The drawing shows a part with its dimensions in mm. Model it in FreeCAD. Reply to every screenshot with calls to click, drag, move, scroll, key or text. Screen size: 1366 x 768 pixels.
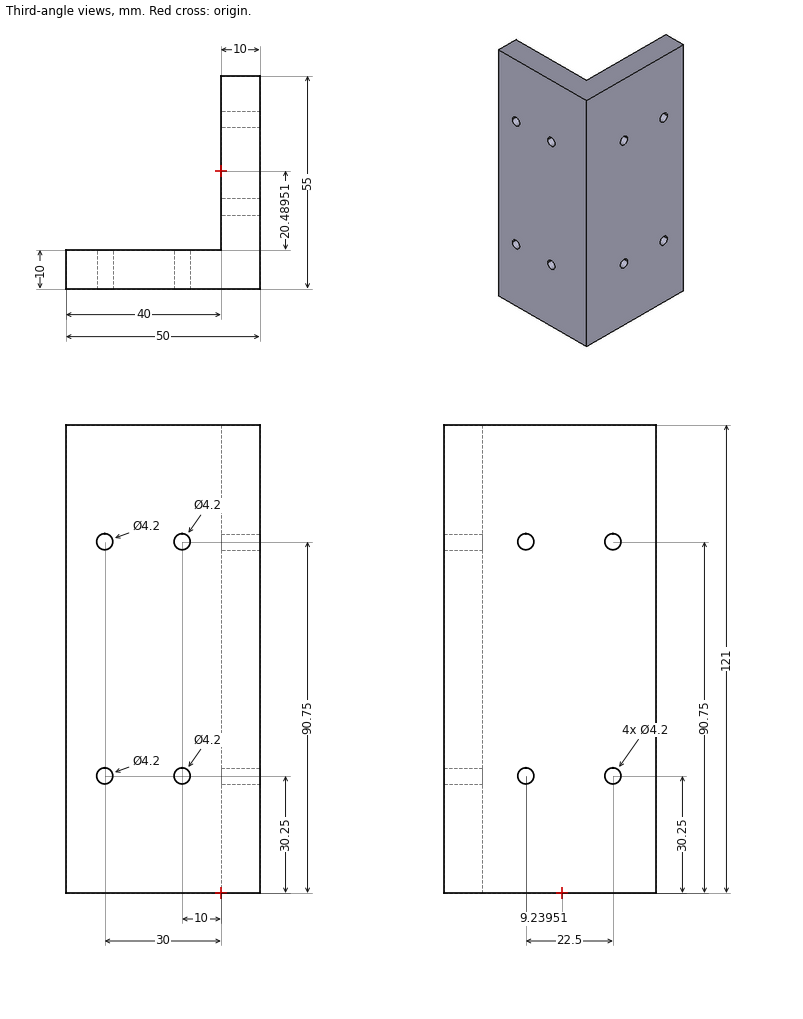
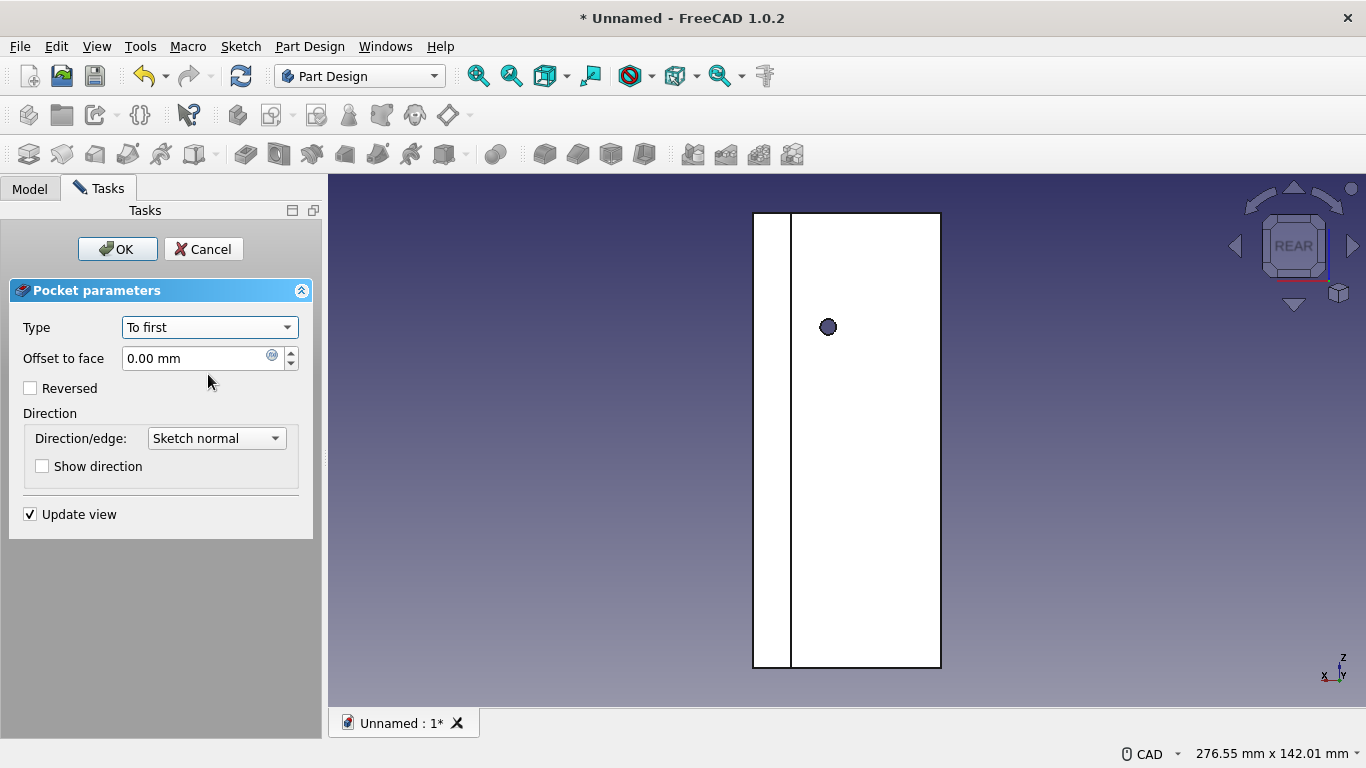
click(118, 249)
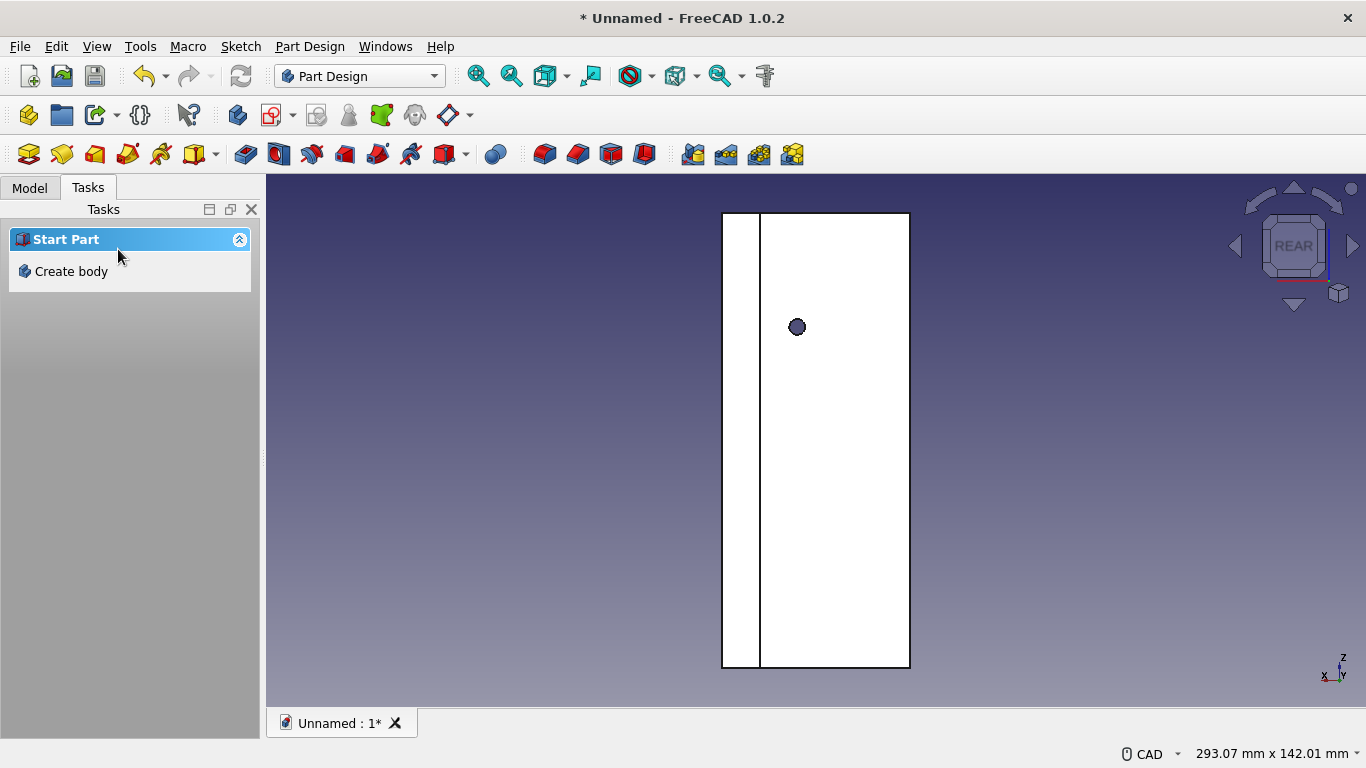
click(835, 439)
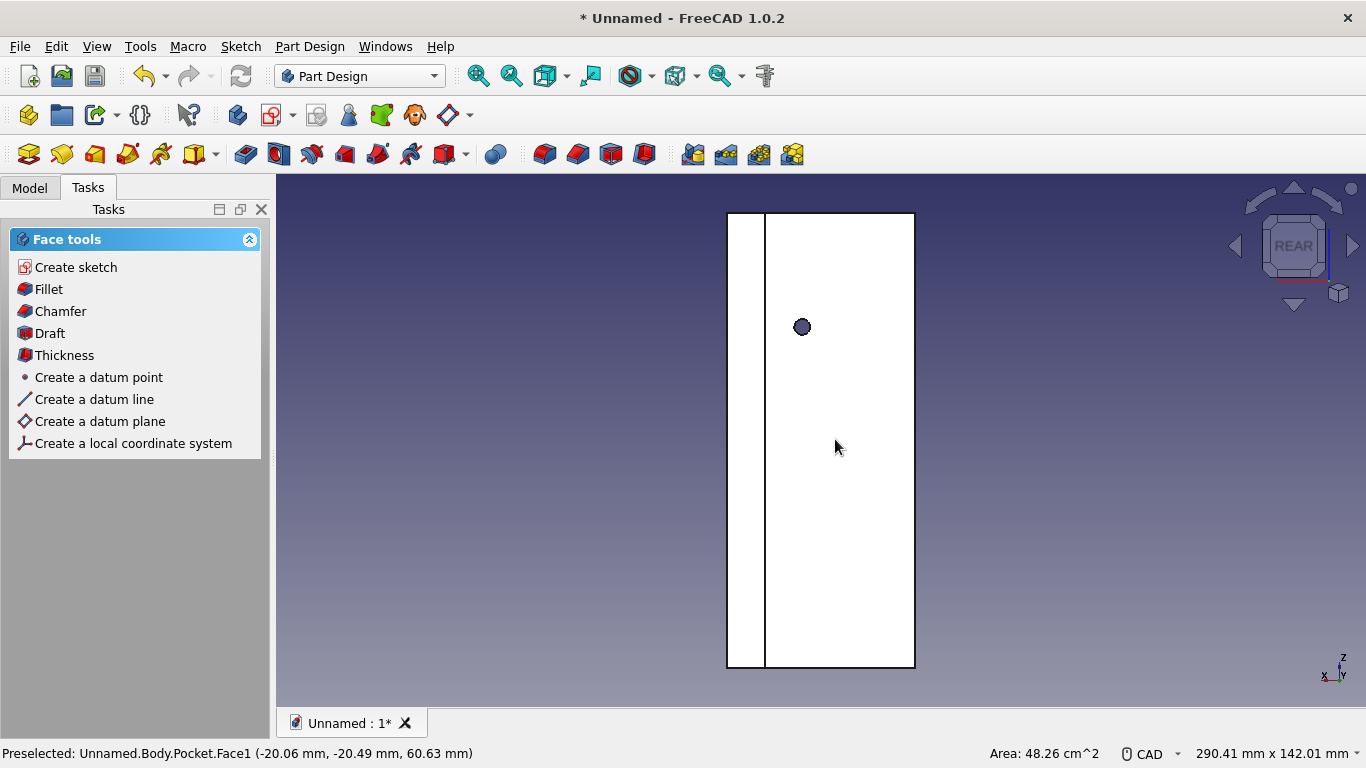
click(270, 116)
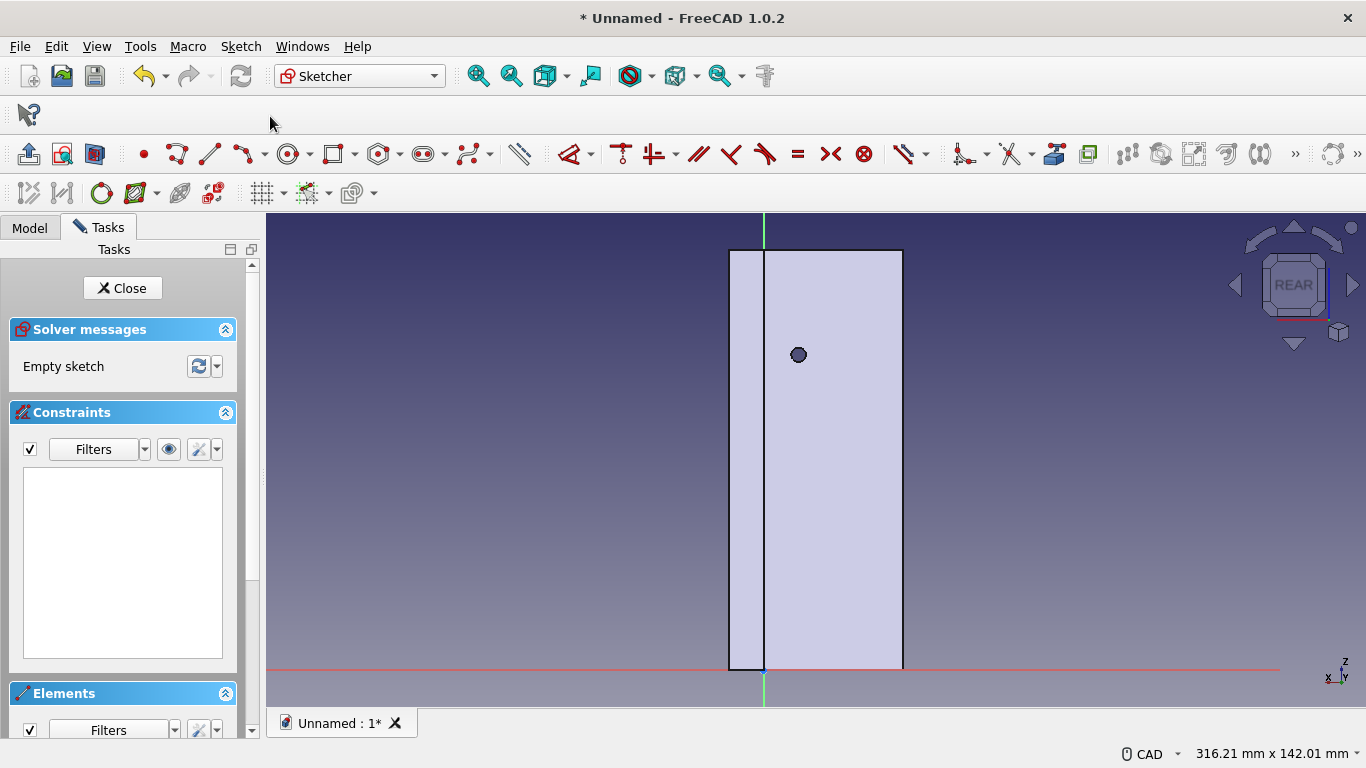
click(95, 154)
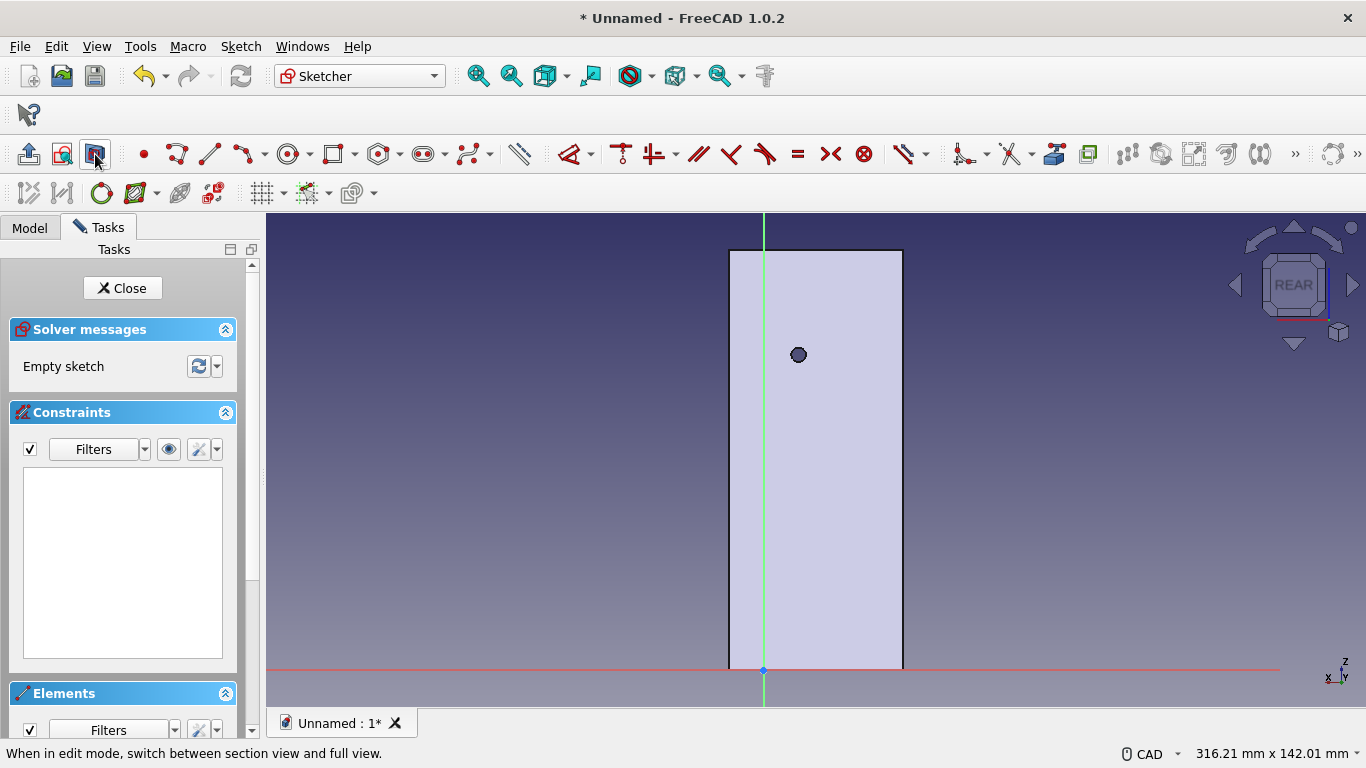
scroll(875, 349, up, 15)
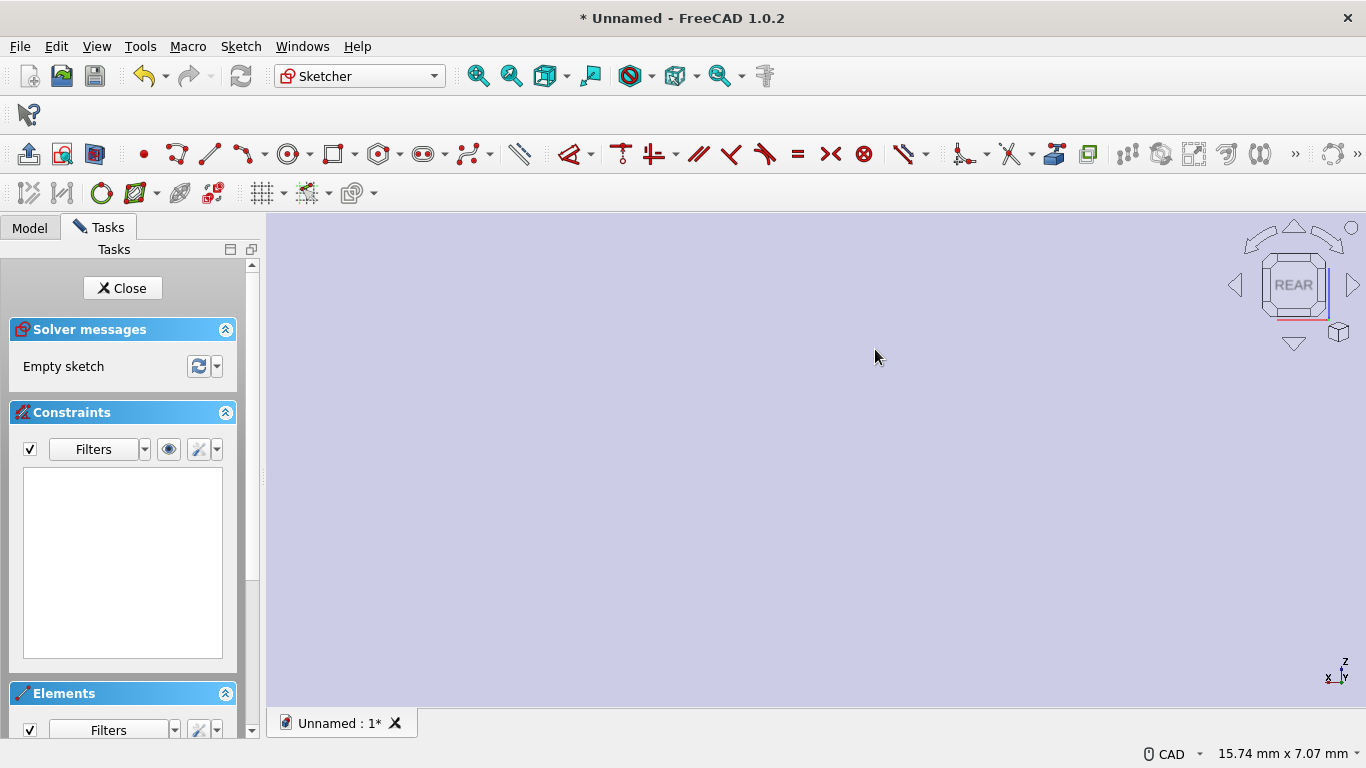
key(g)
key(c)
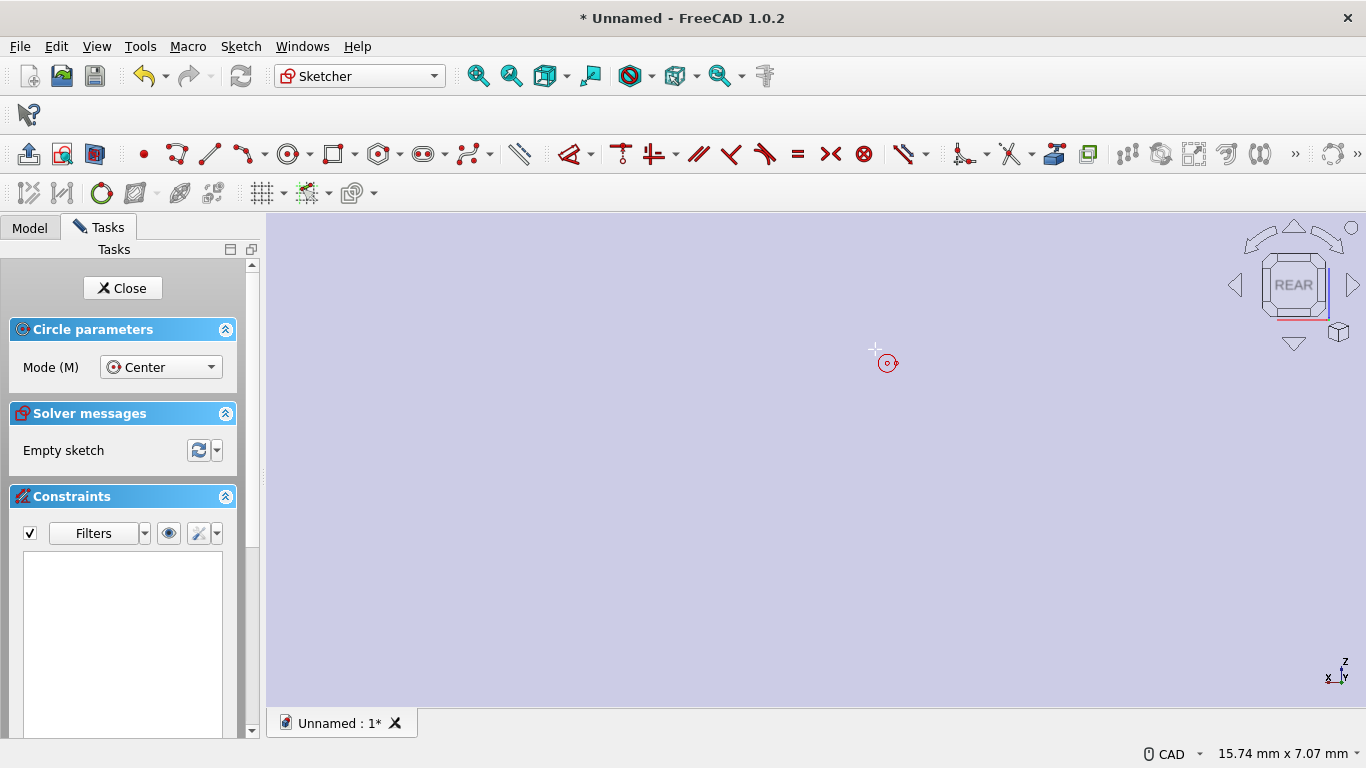
click(727, 460)
move(831, 356)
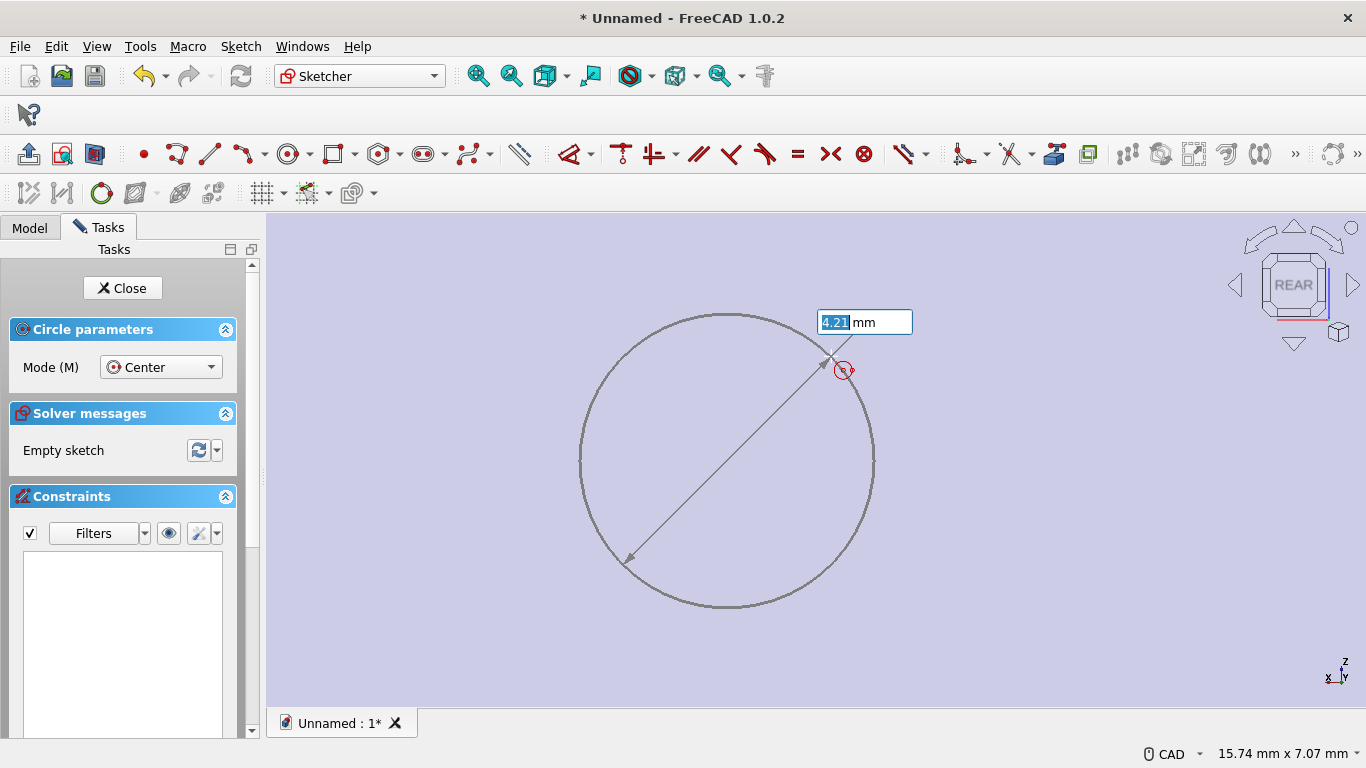
text(4.2)
key(Return)
key(Escape)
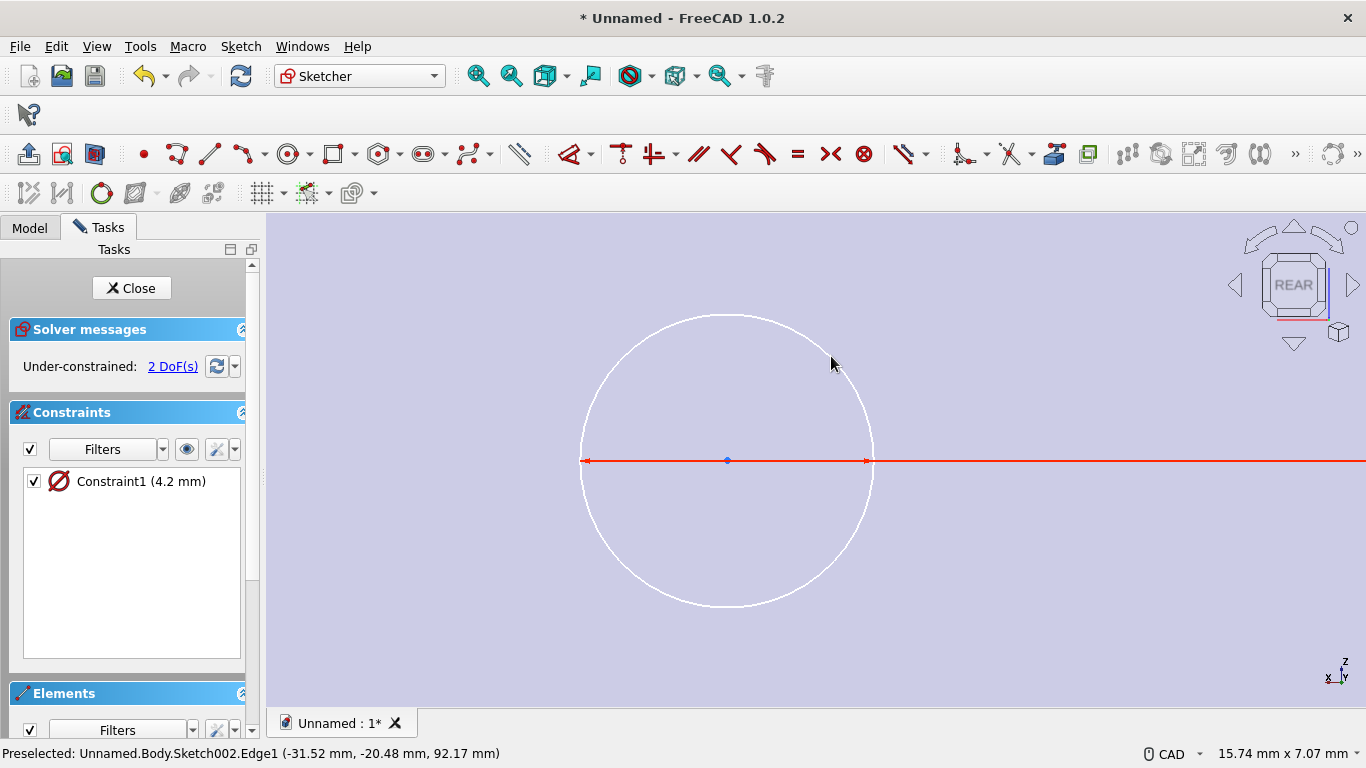
click(568, 154)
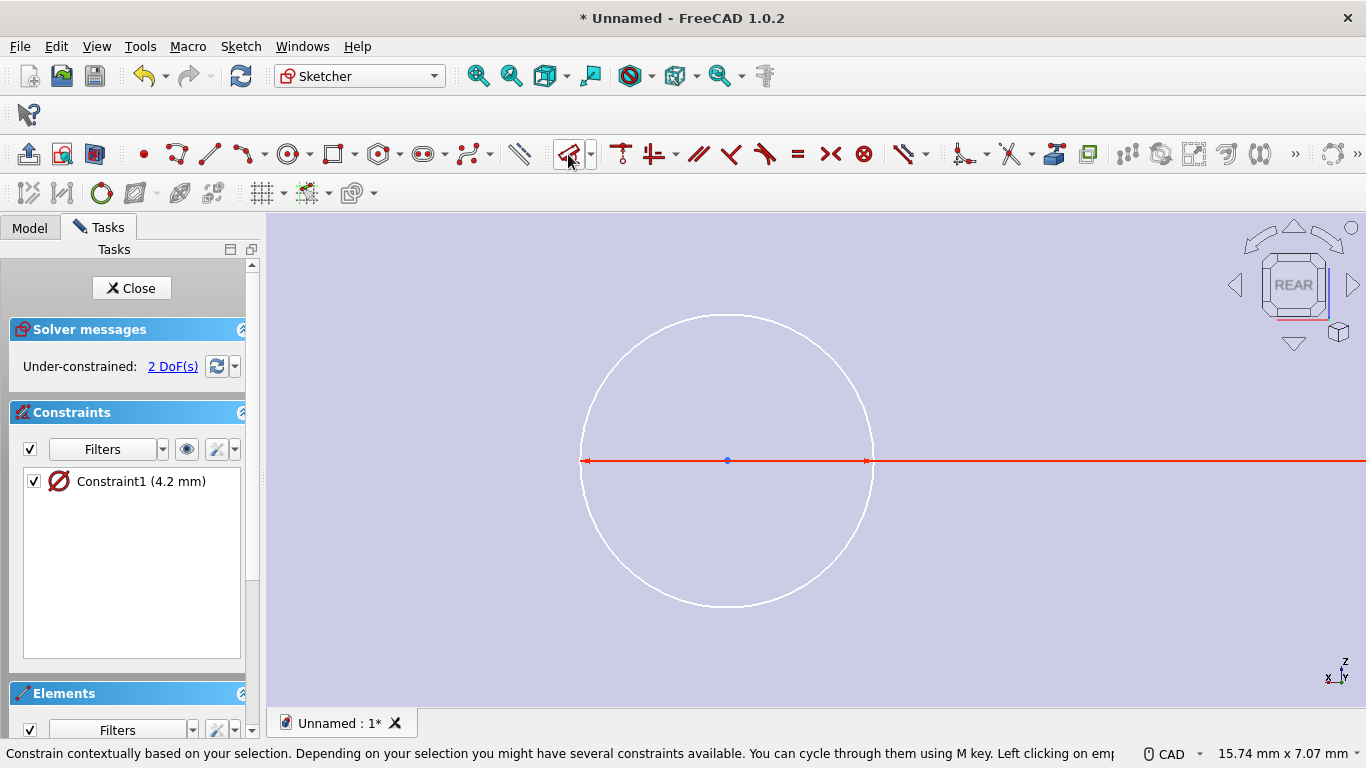
click(727, 461)
click(511, 427)